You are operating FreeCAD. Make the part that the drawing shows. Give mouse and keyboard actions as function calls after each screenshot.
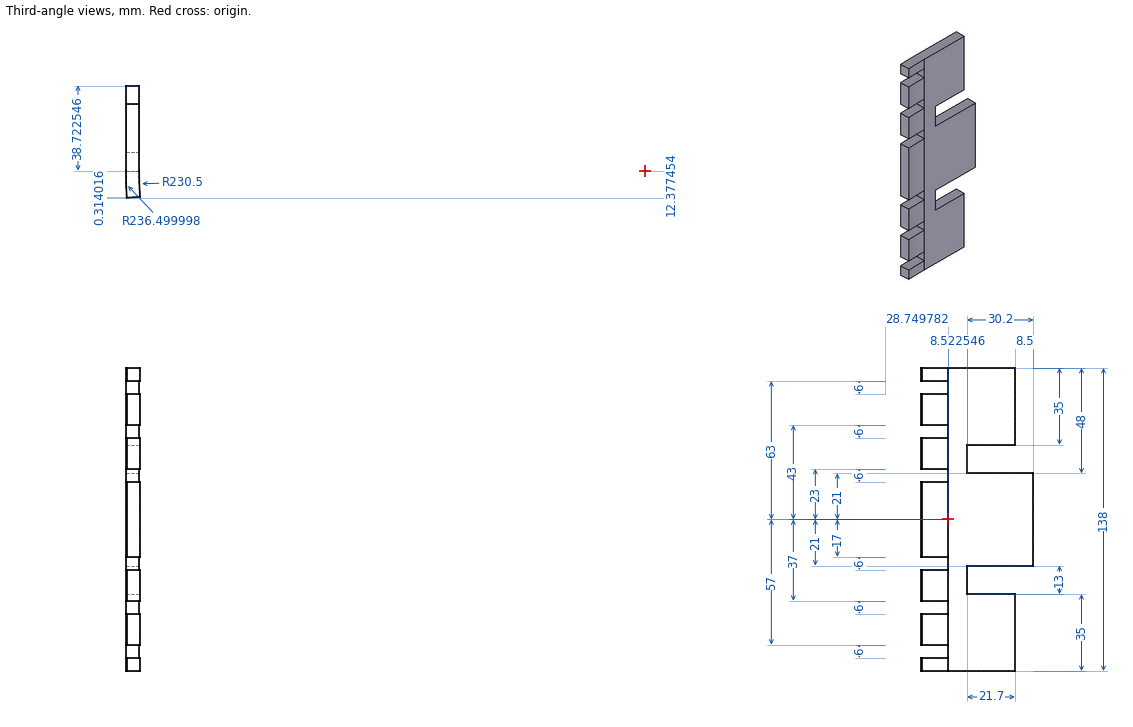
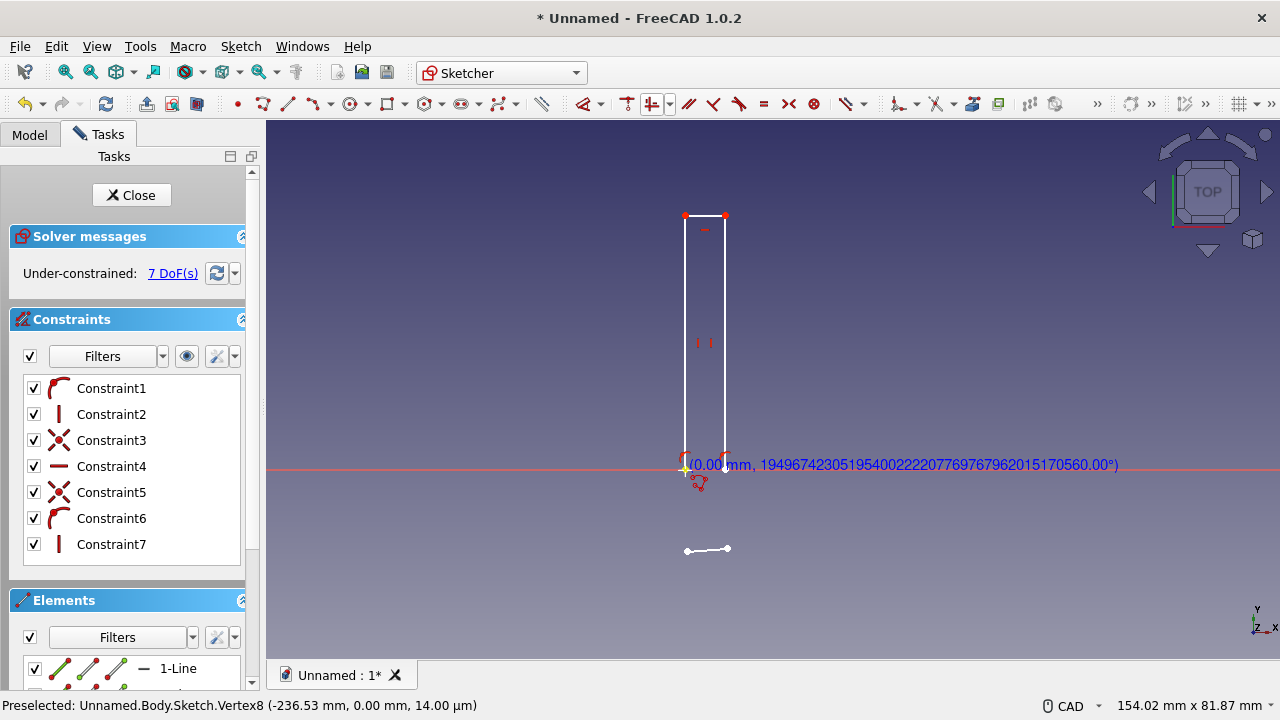
key(g)
key(3)
key(a)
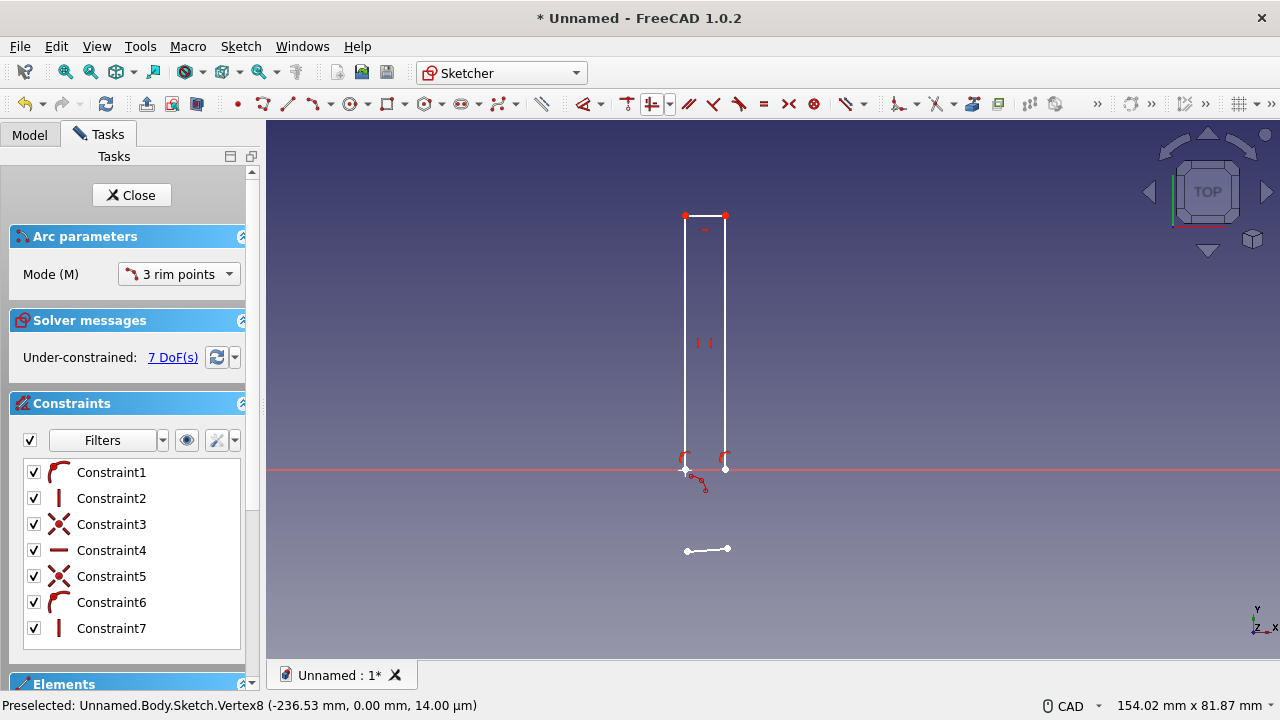
click(727, 549)
click(725, 470)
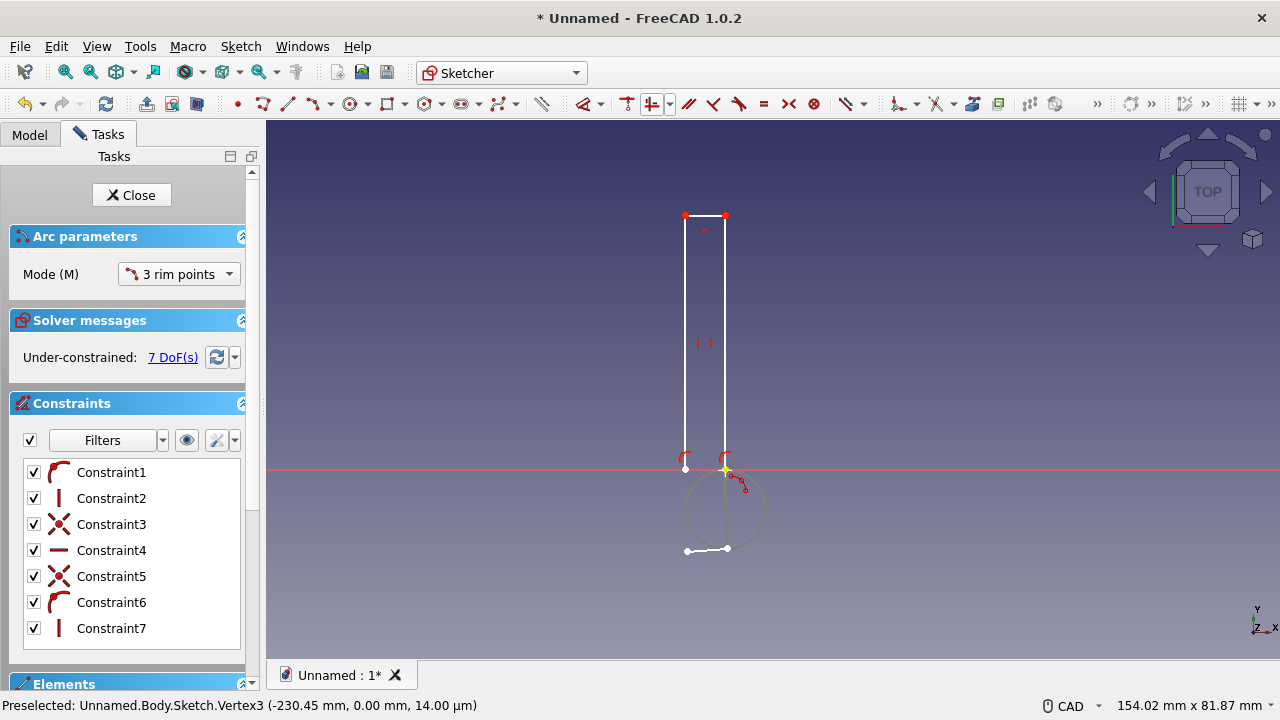
scroll(725, 509, up, 18)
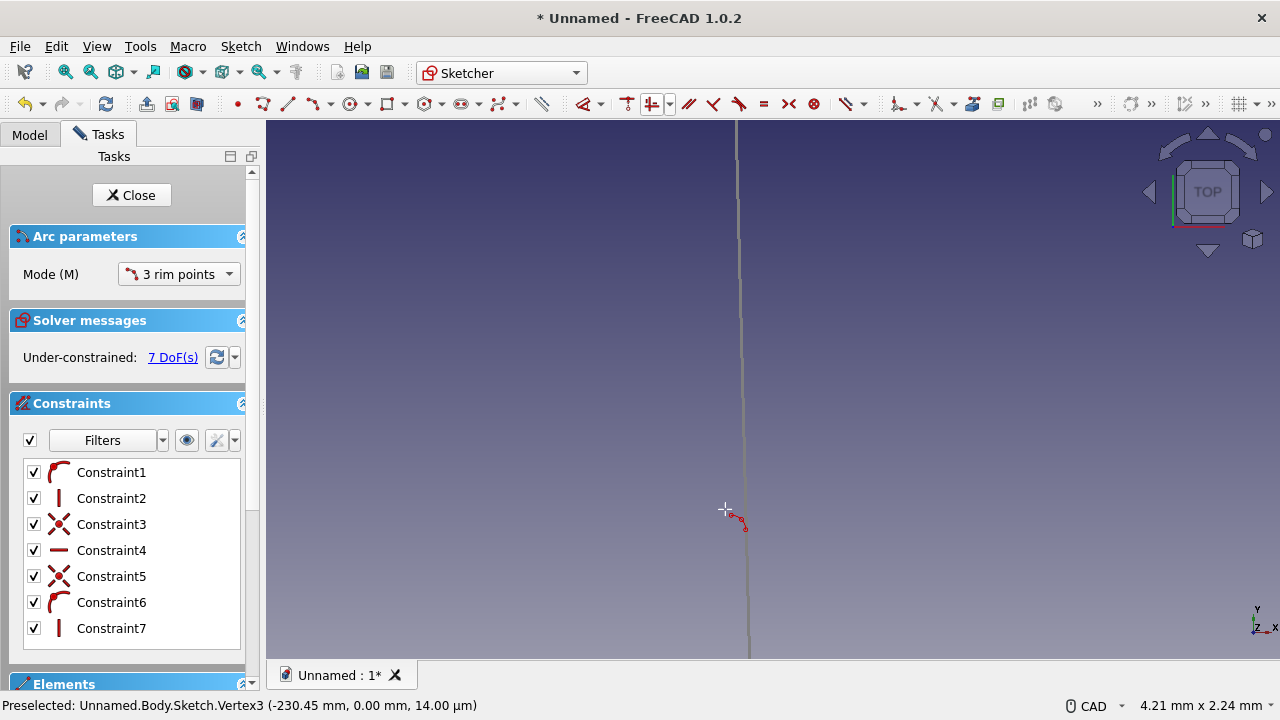
click(716, 498)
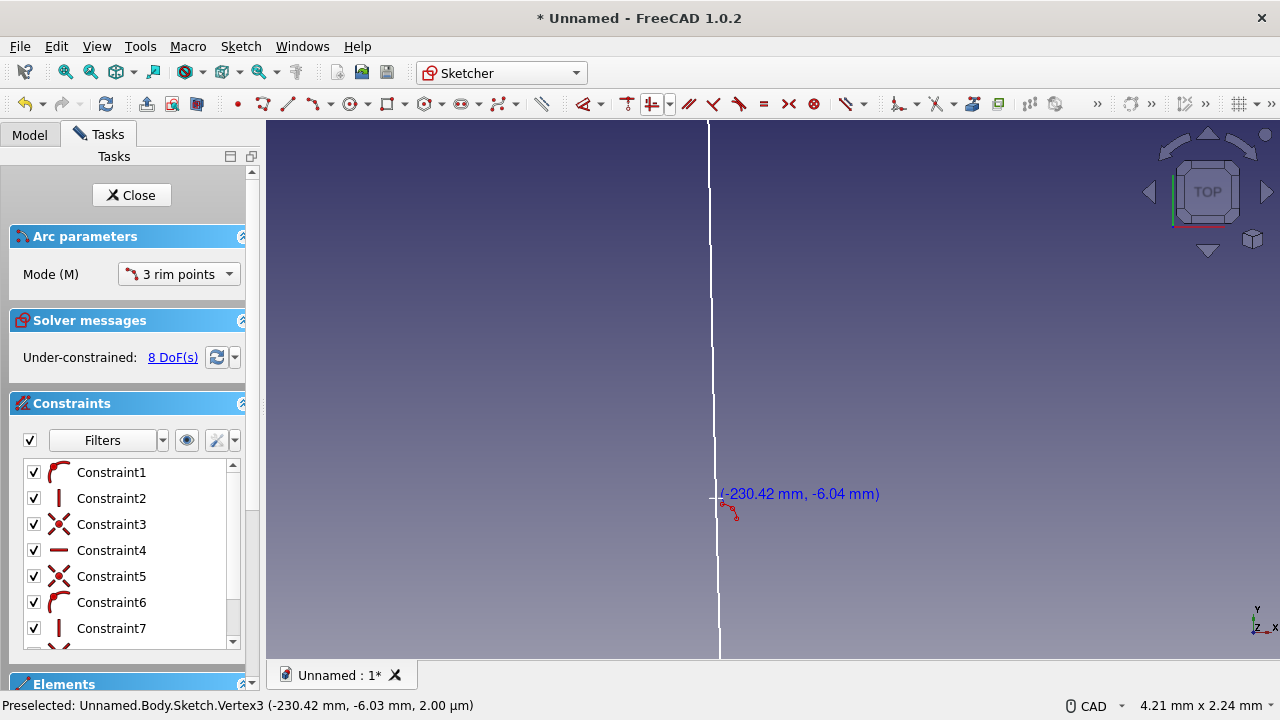
scroll(728, 546, down, 17)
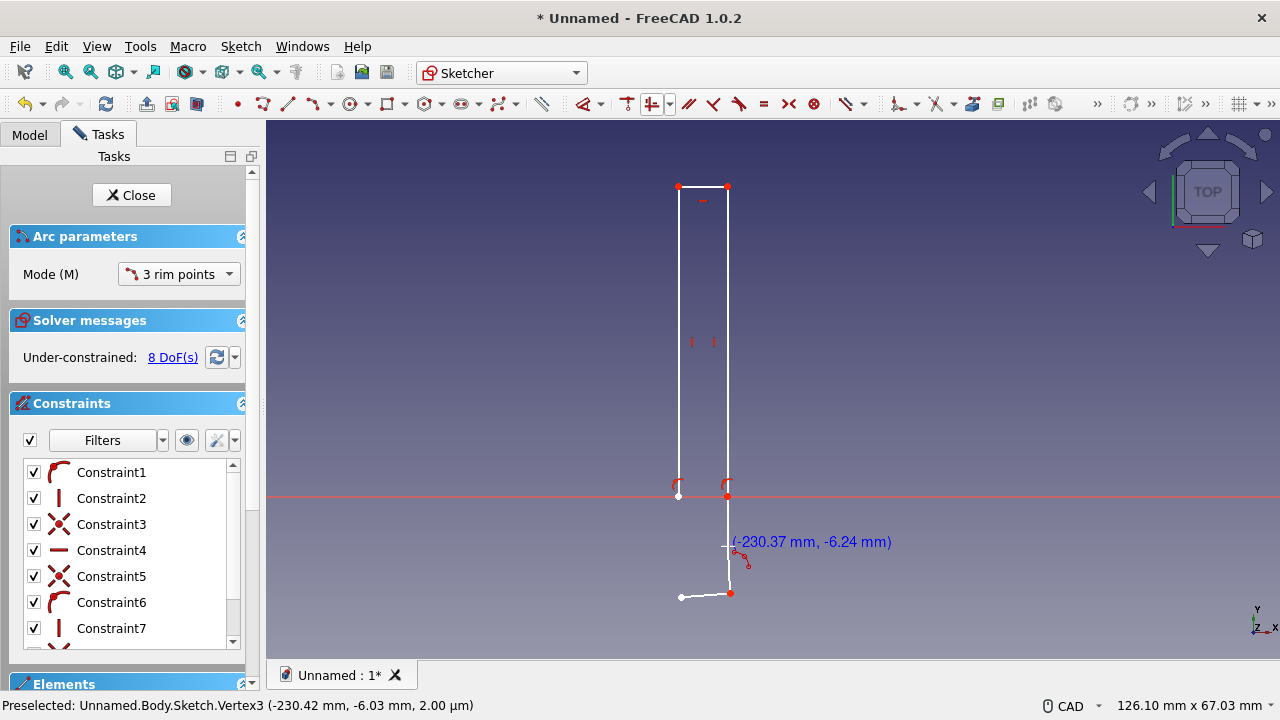
click(679, 497)
click(681, 597)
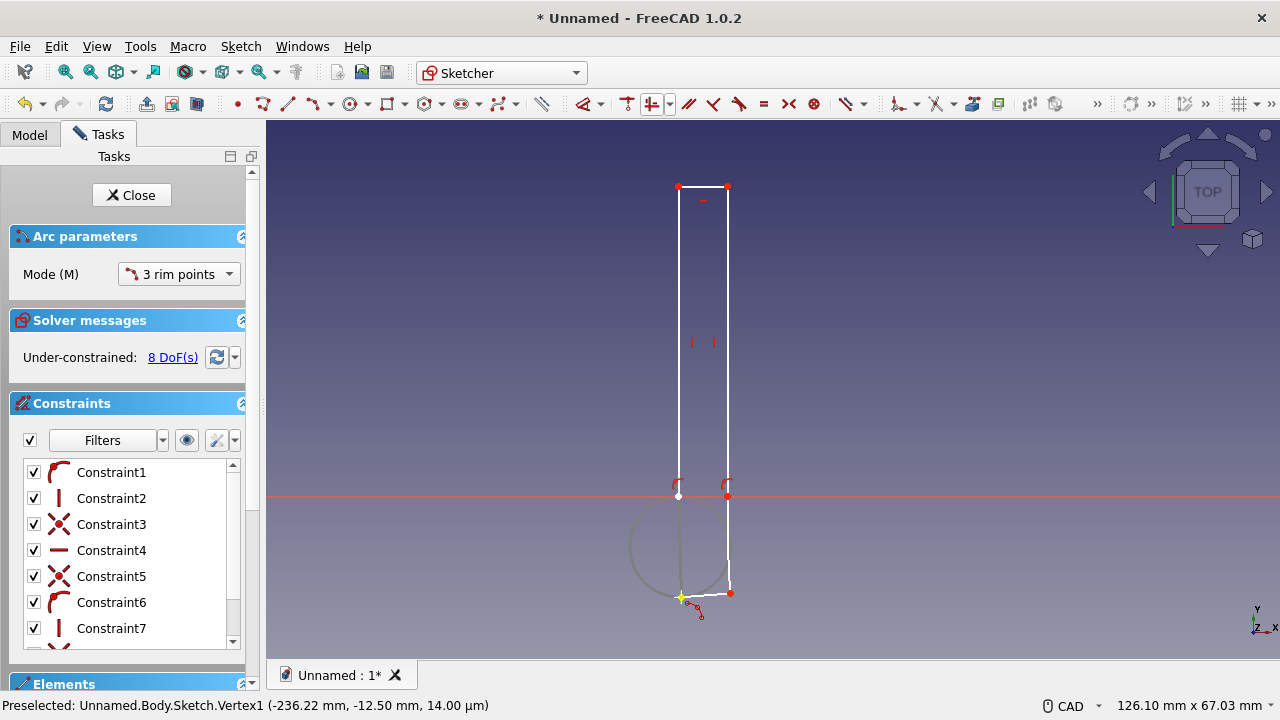
scroll(680, 546, up, 16)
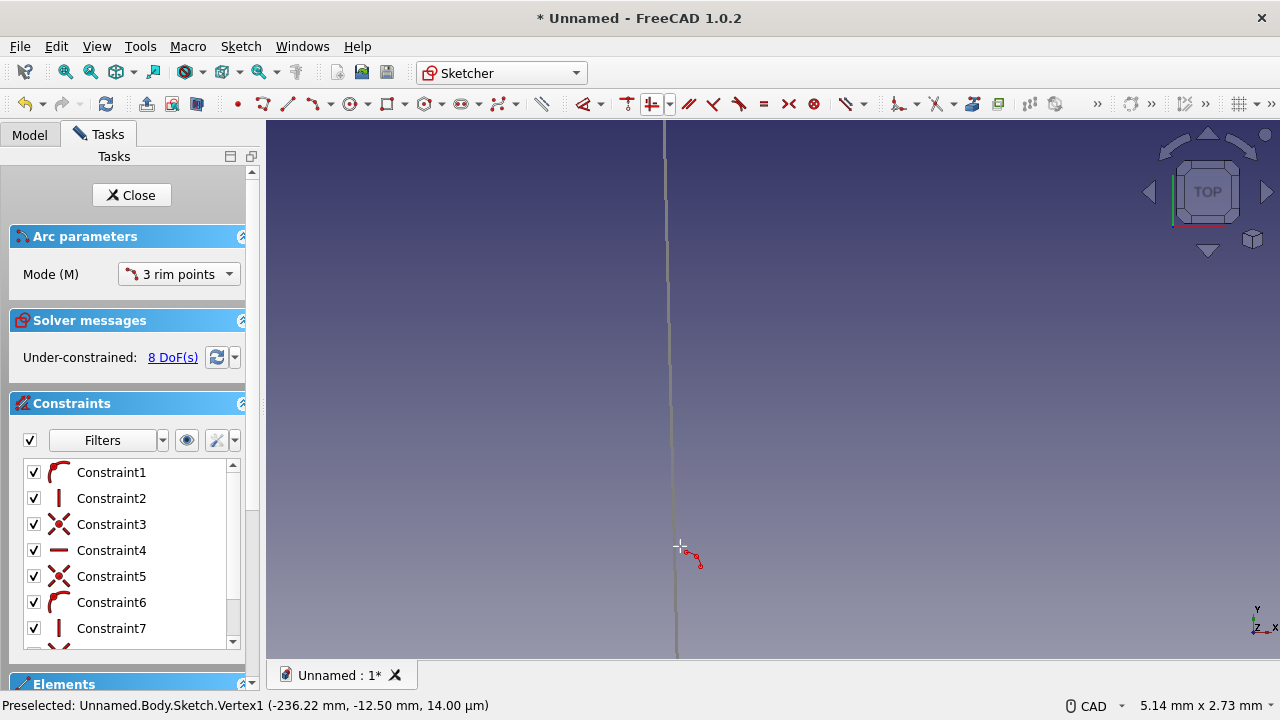
click(666, 538)
key(Escape)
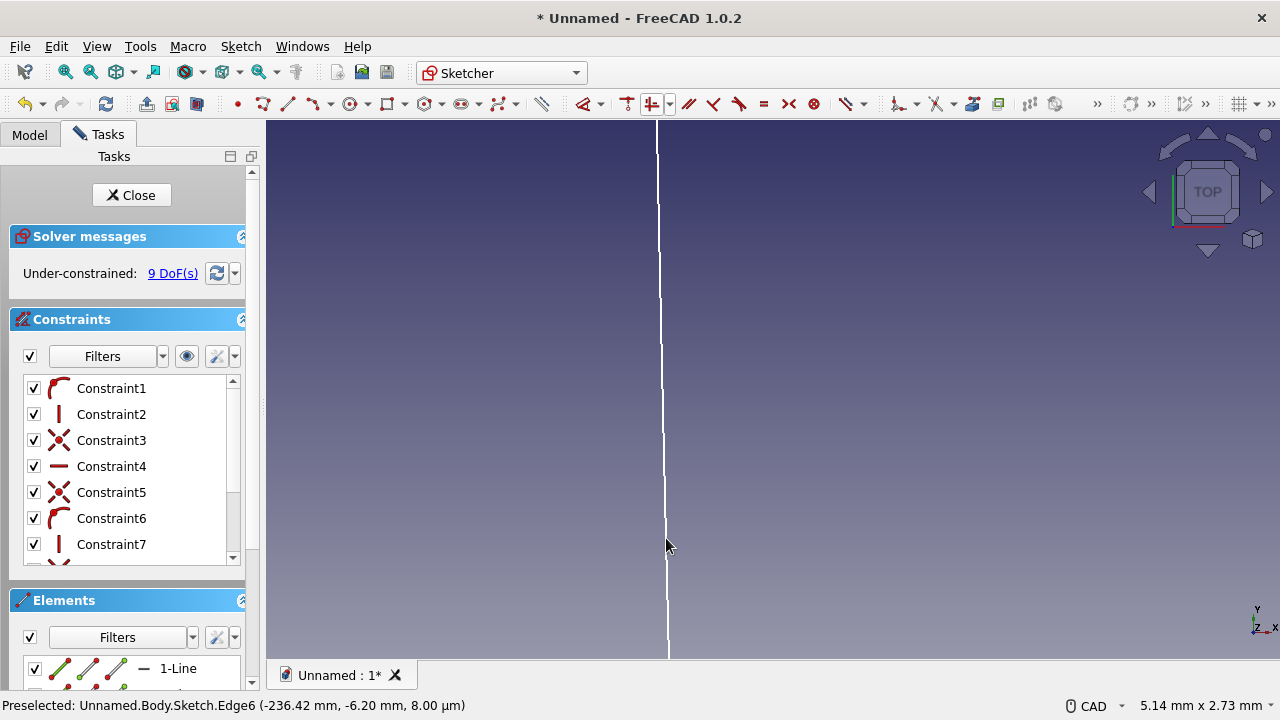
scroll(680, 546, down, 16)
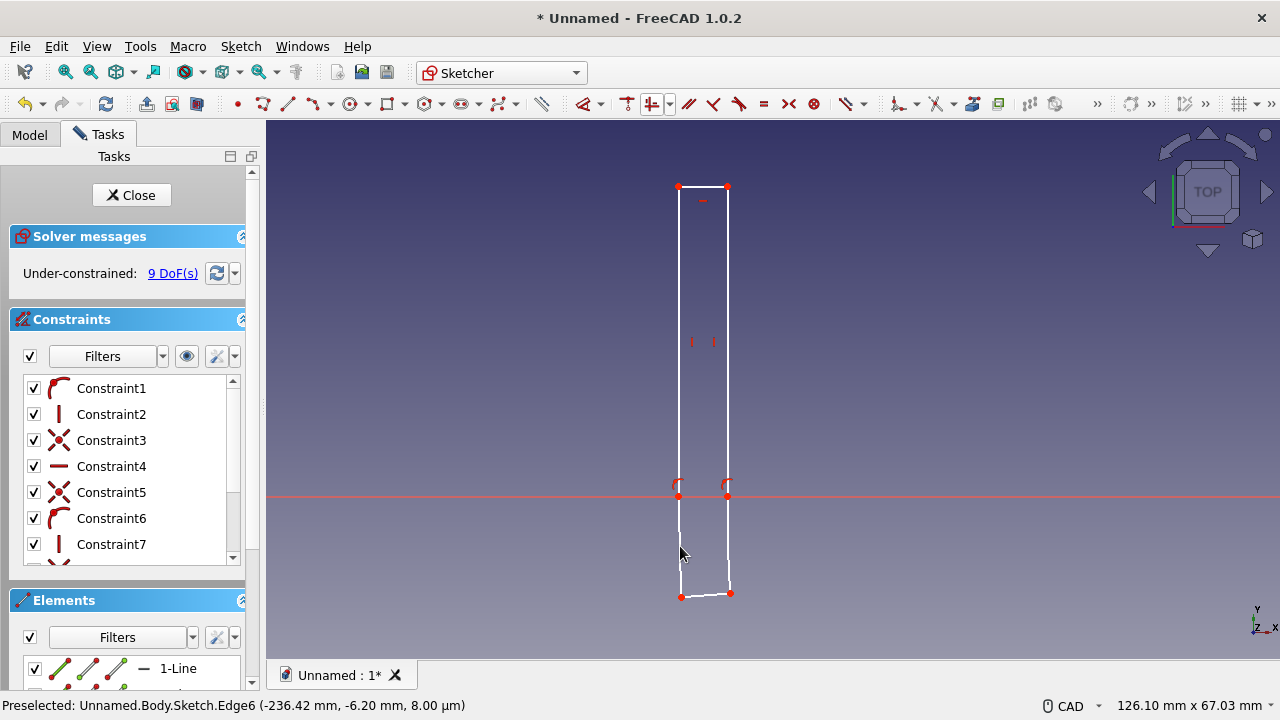
click(728, 526)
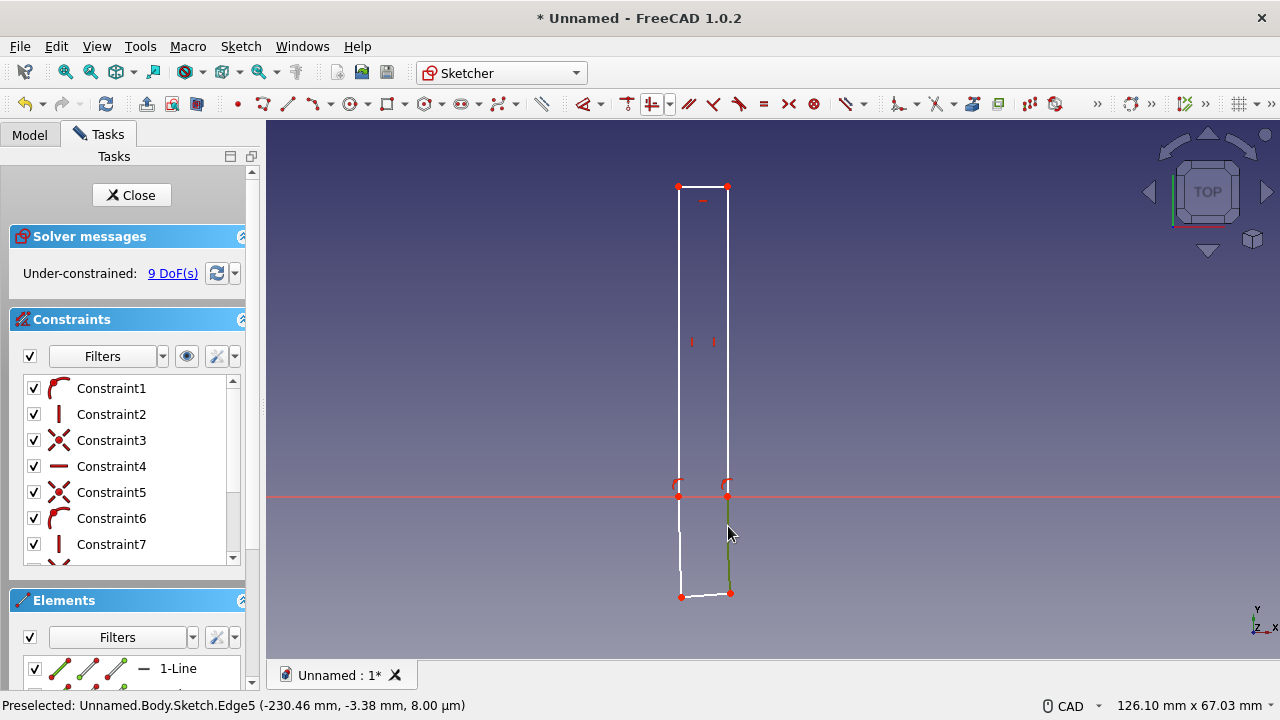
click(679, 527)